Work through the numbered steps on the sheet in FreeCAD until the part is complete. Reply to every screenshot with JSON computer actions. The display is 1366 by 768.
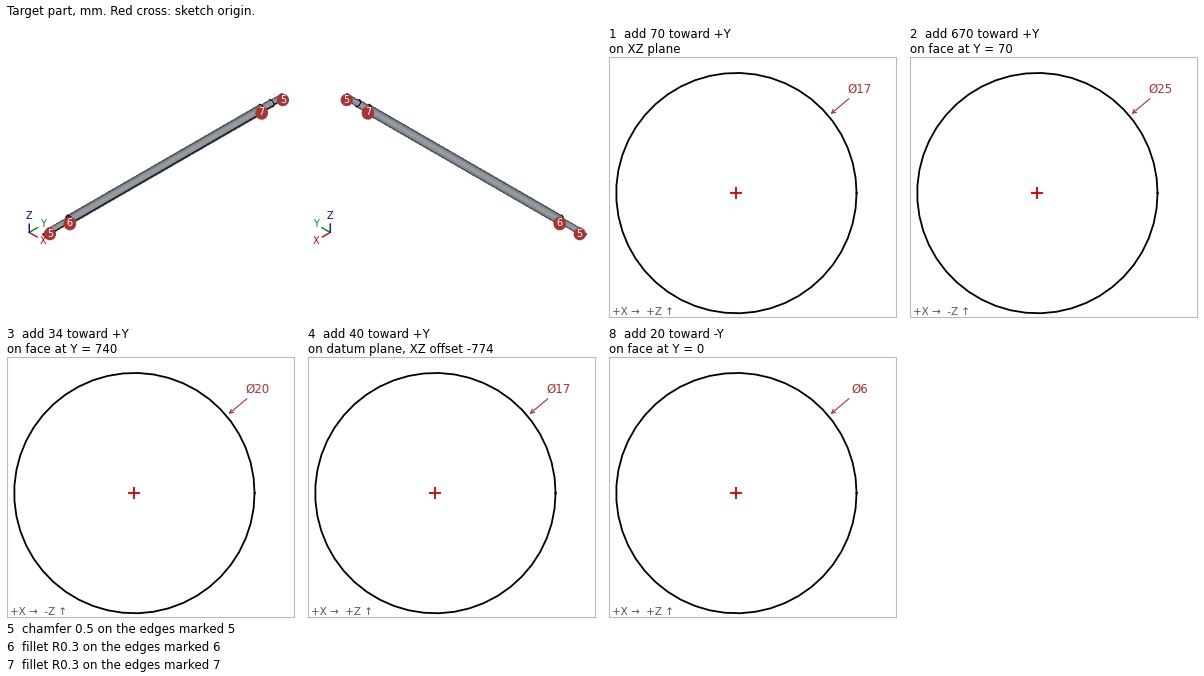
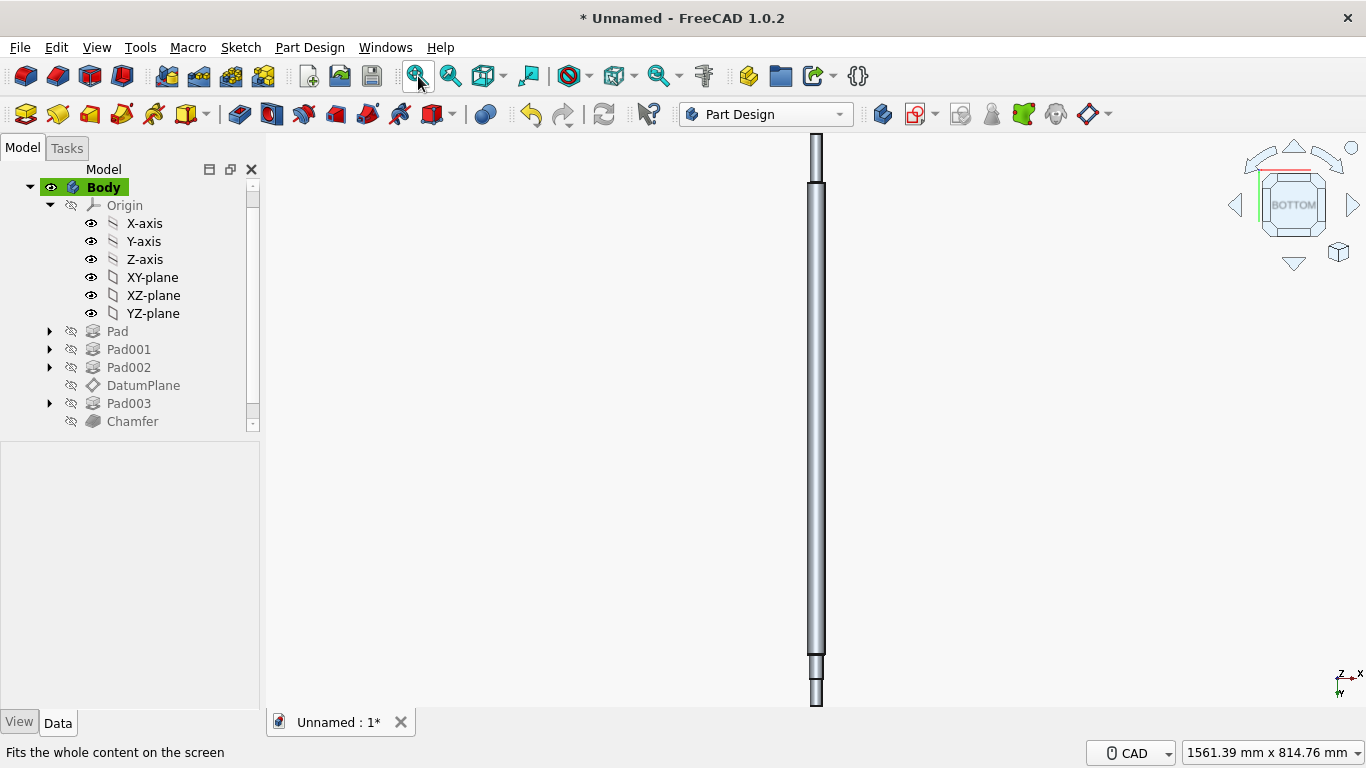
{"action": "left_click", "coordinate": [418, 76]}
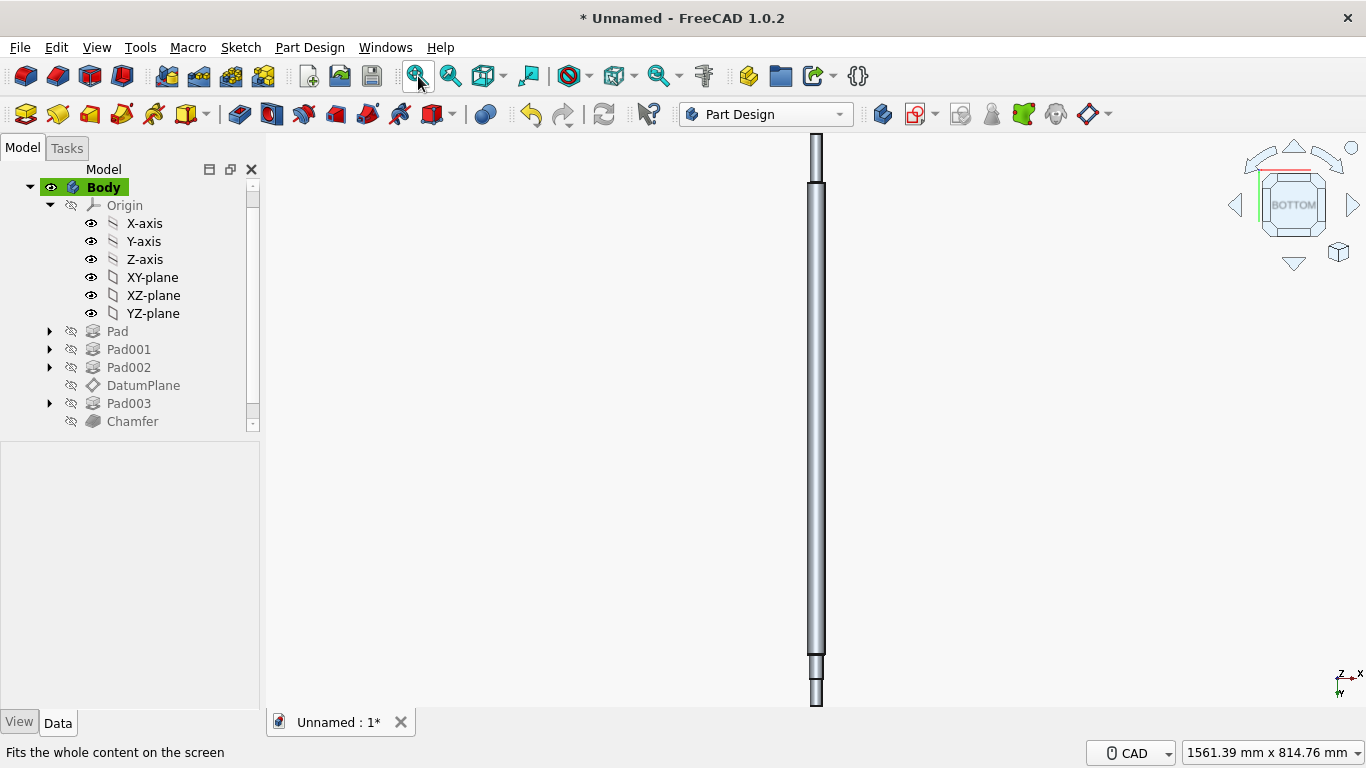
{"action": "key", "text": "4"}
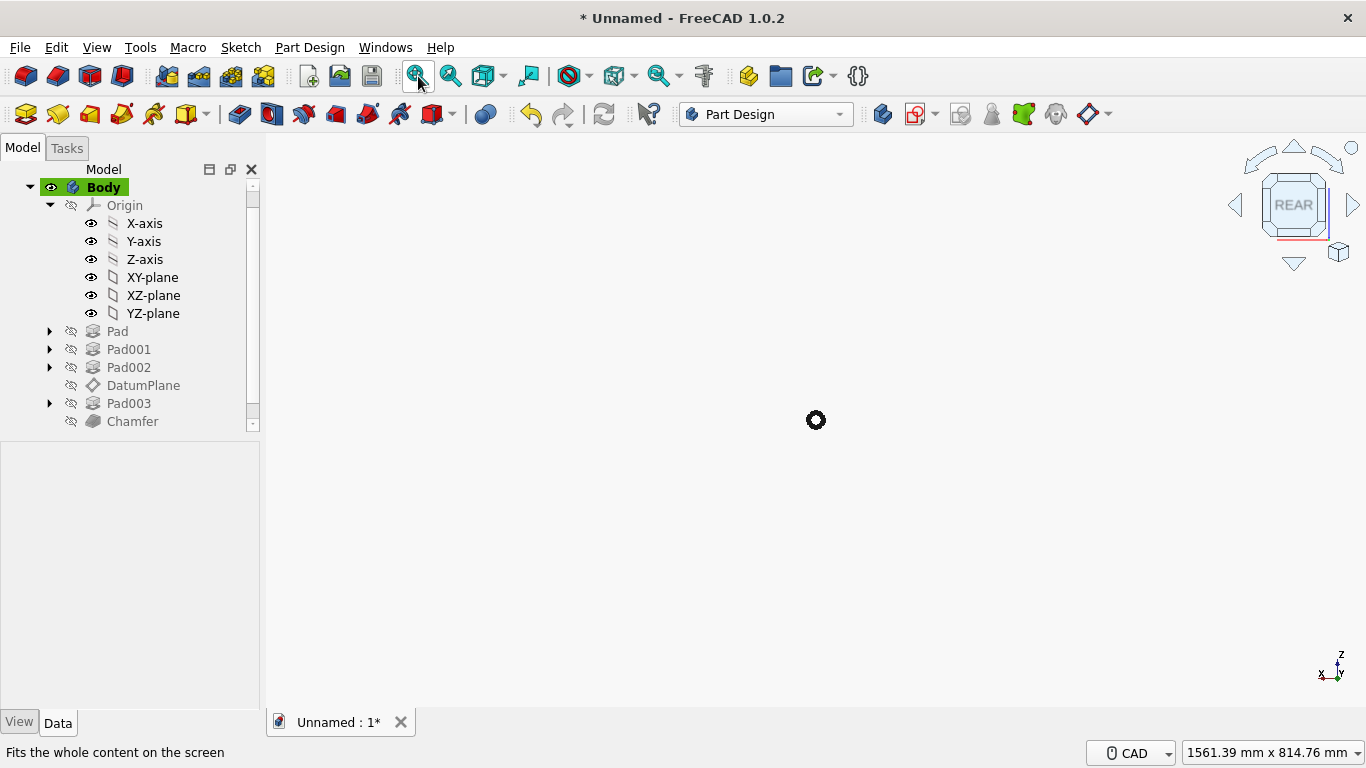
{"action": "left_click", "coordinate": [418, 76]}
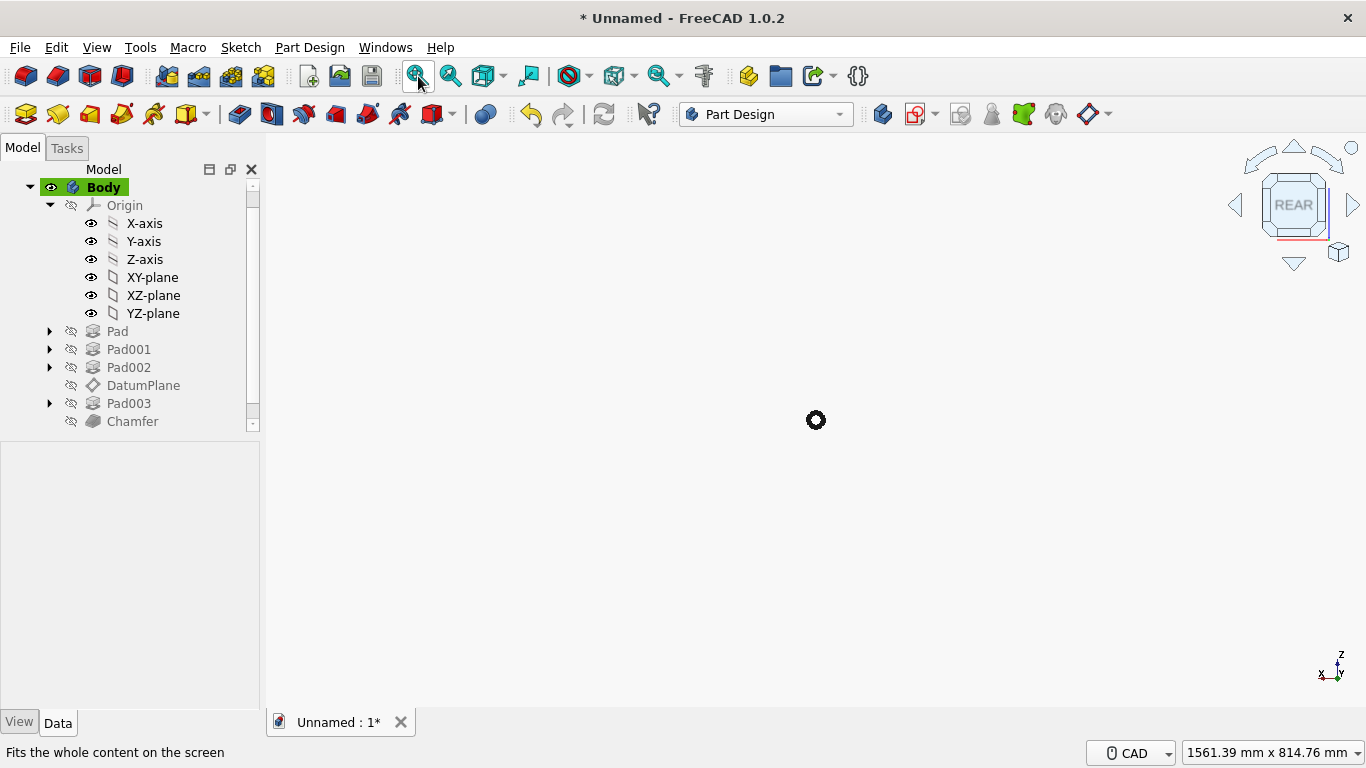
{"action": "key", "text": "6"}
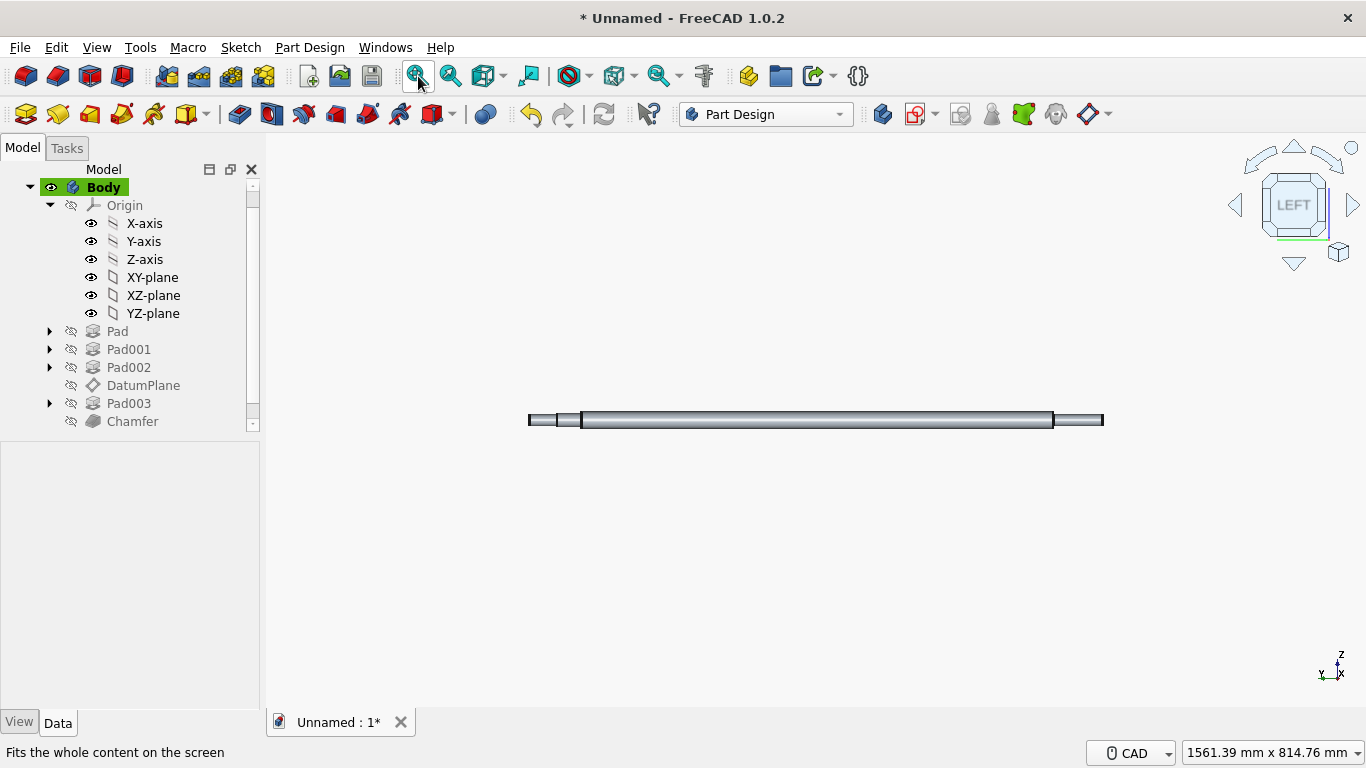
{"action": "key", "text": "v 3"}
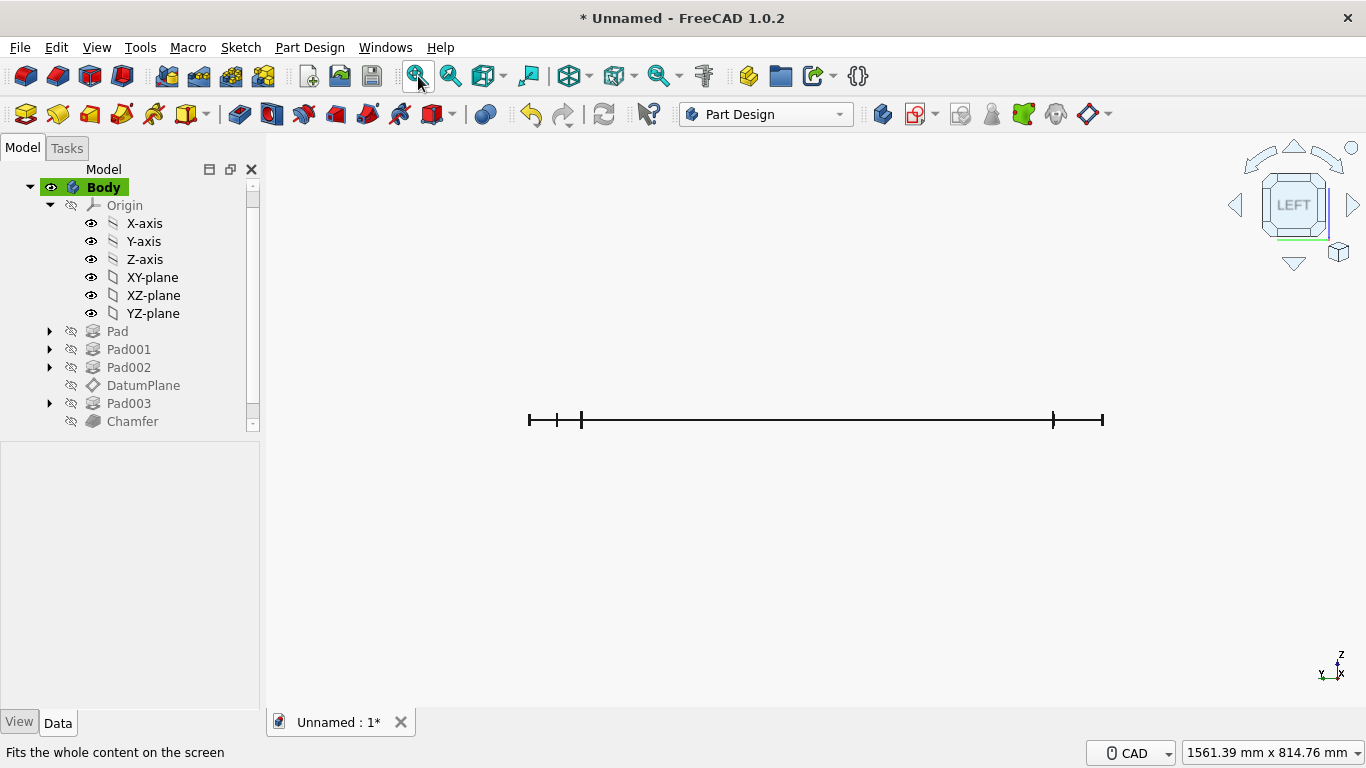
{"action": "key", "text": "0"}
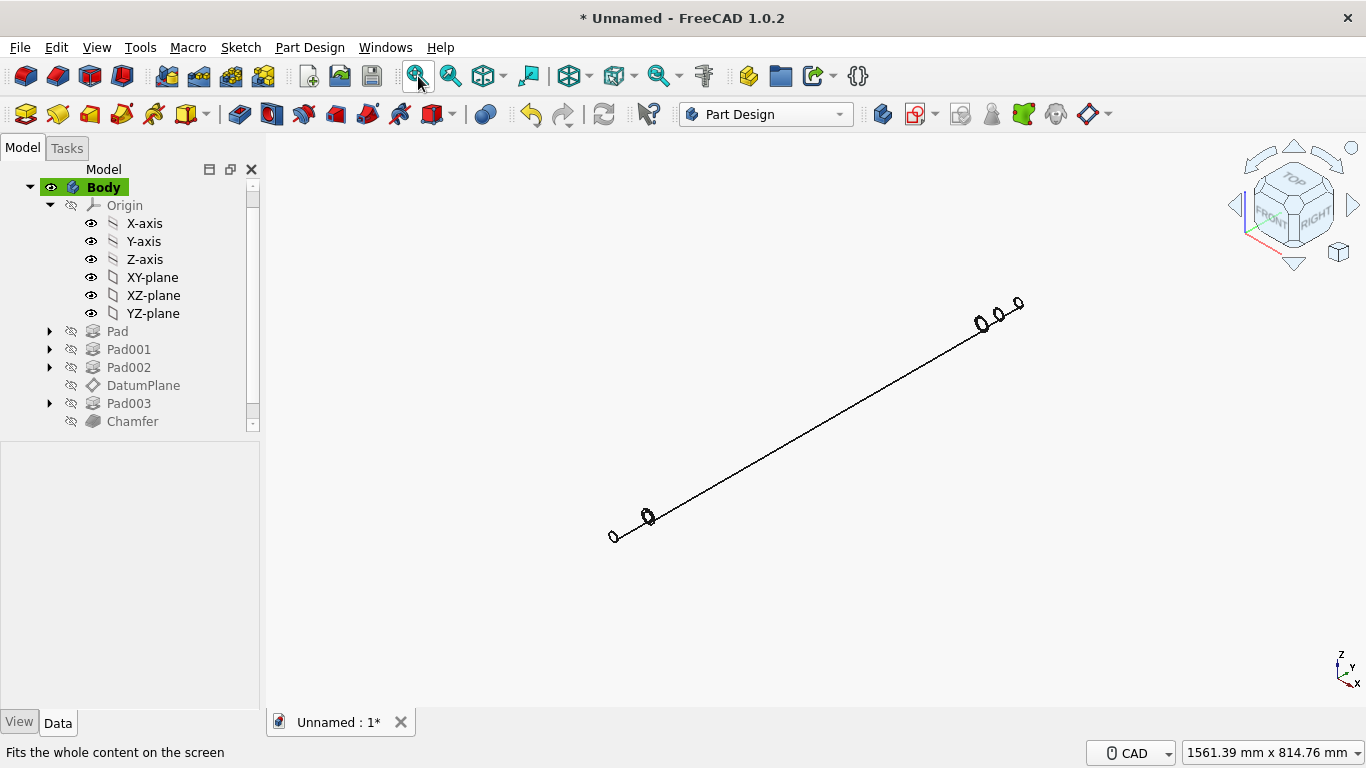
{"action": "left_click", "coordinate": [418, 76]}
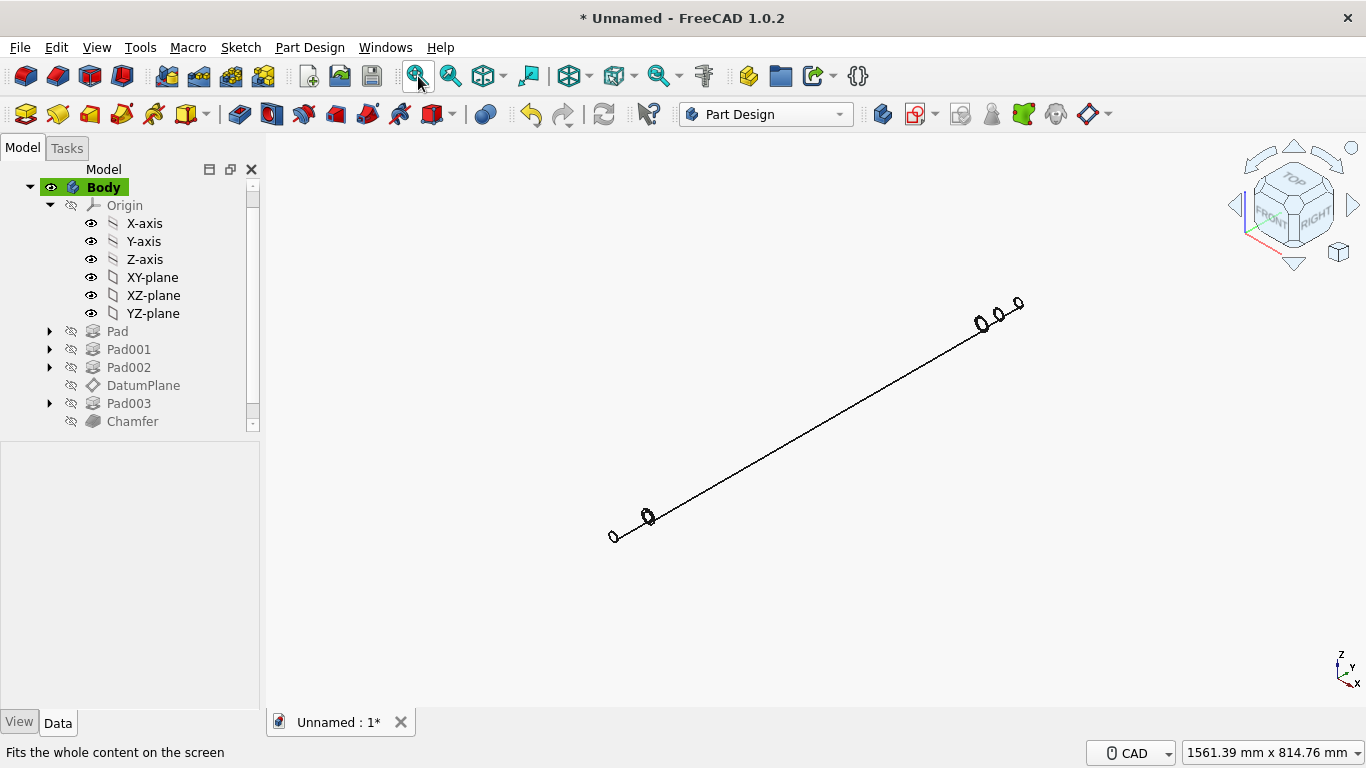
{"action": "left_click", "coordinate": [978, 324]}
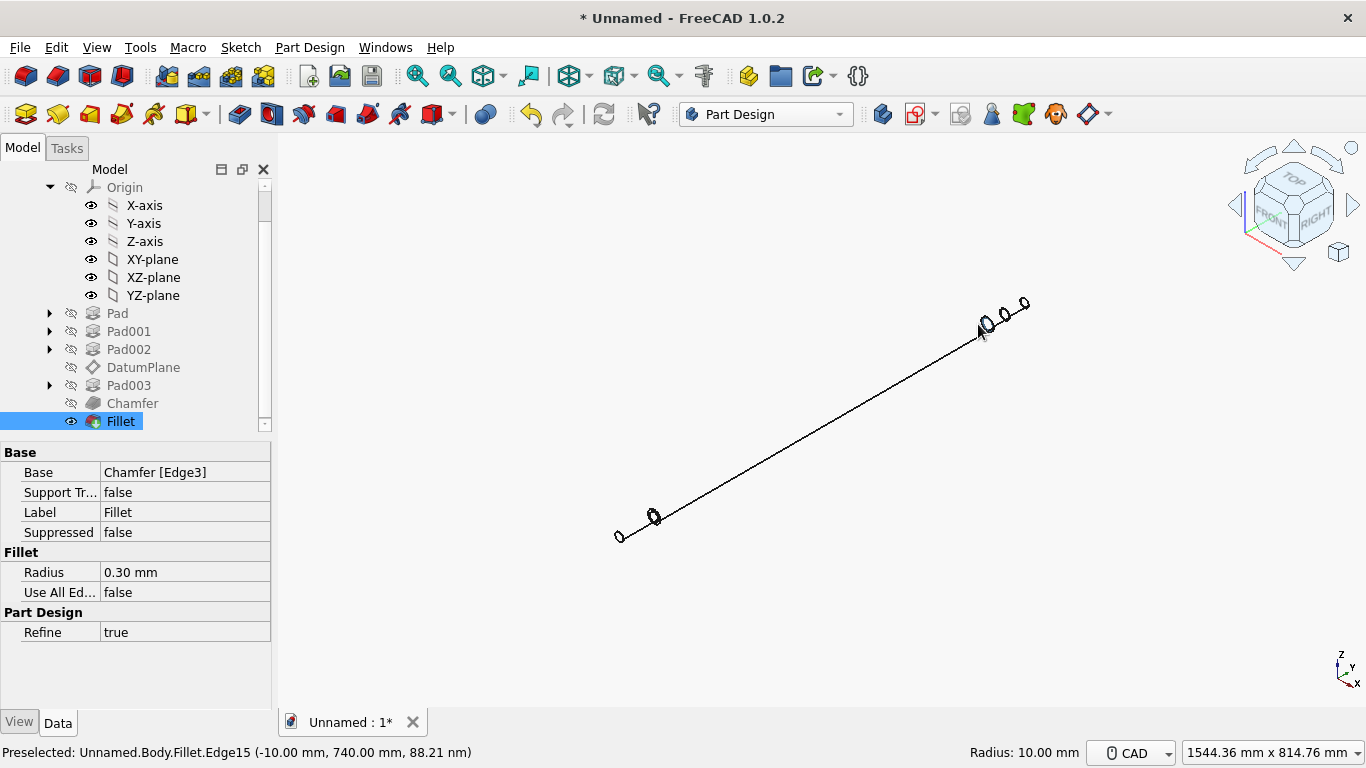
{"action": "key", "text": "v 1"}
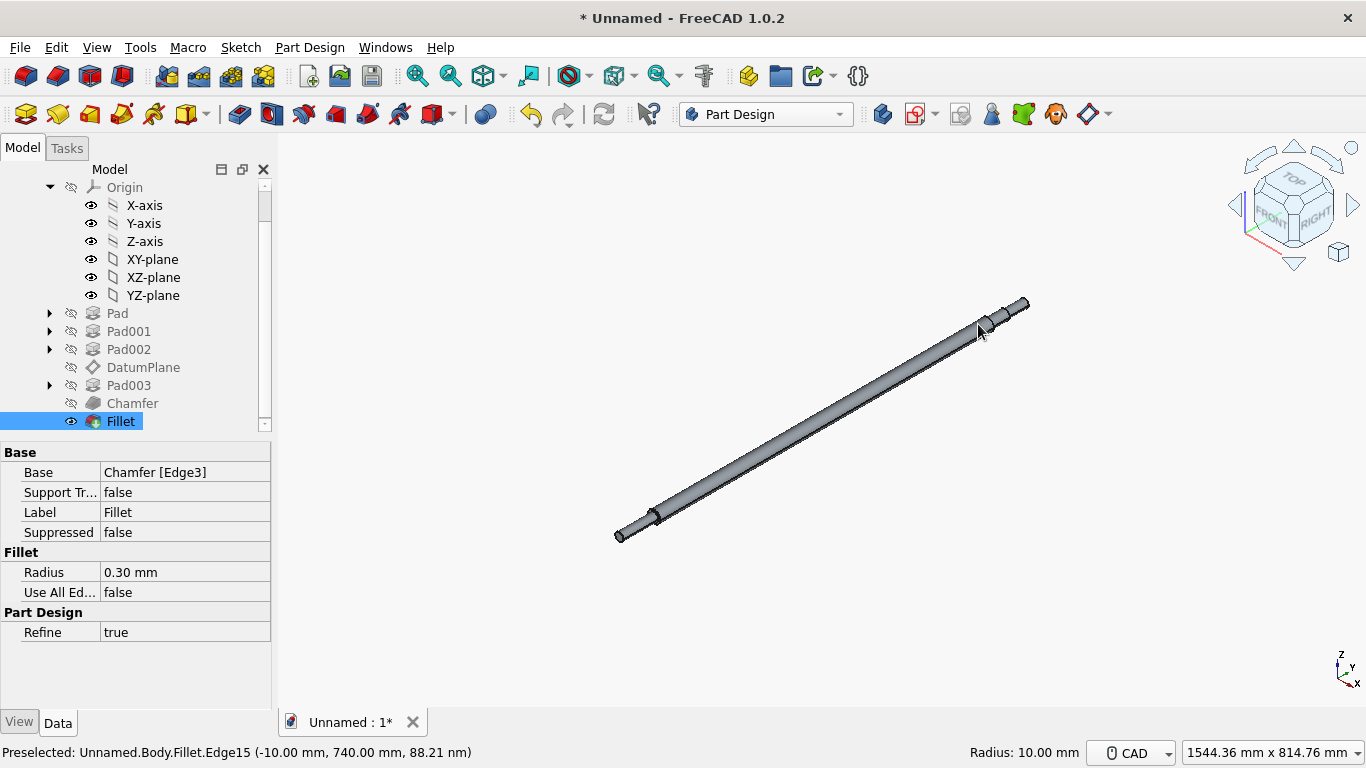
{"action": "left_click", "coordinate": [26, 76]}